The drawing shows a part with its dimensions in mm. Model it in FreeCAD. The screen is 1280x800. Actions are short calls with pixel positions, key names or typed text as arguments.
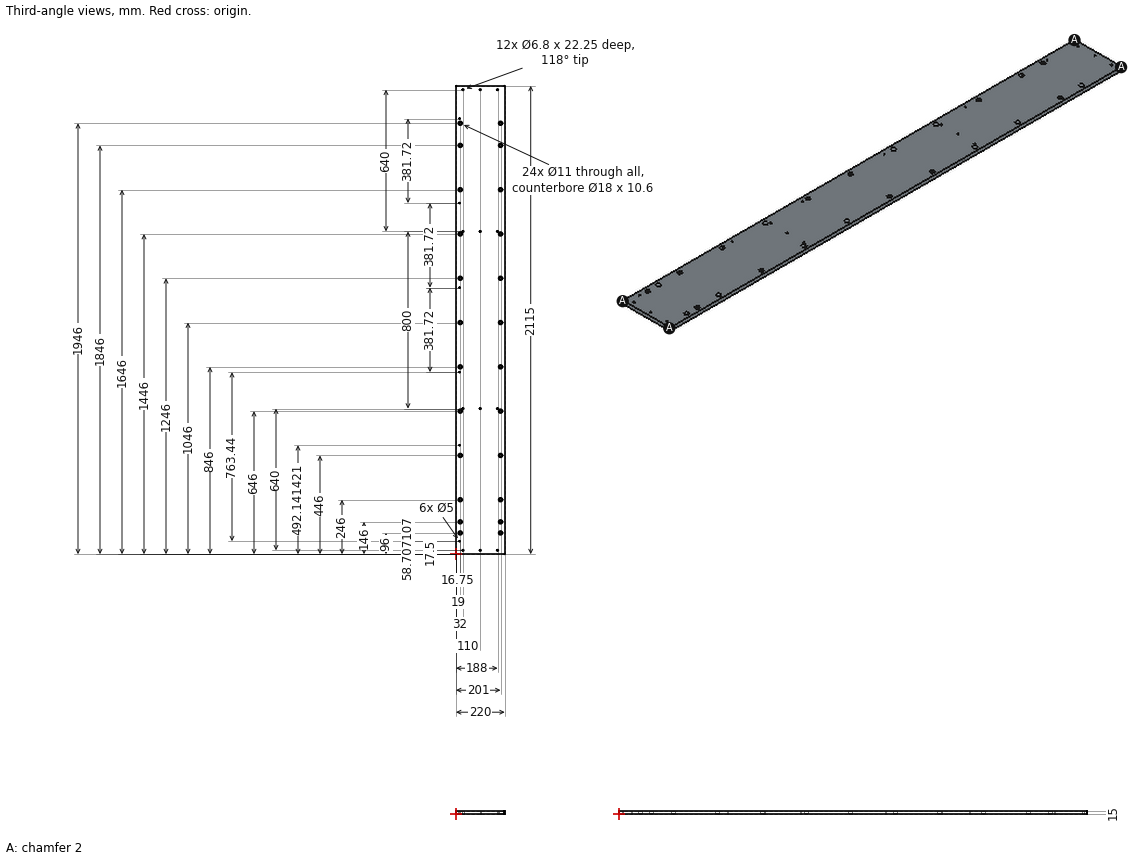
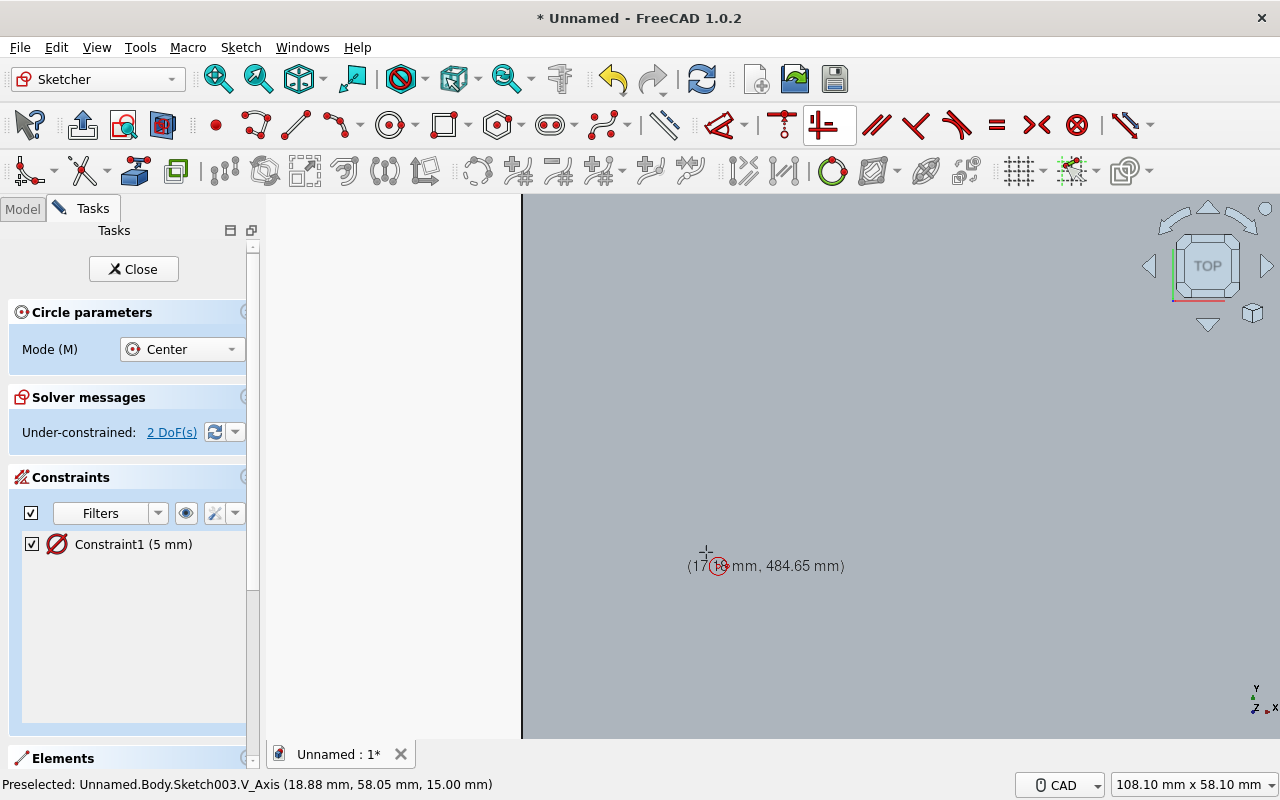
scroll(704, 466, down, 15)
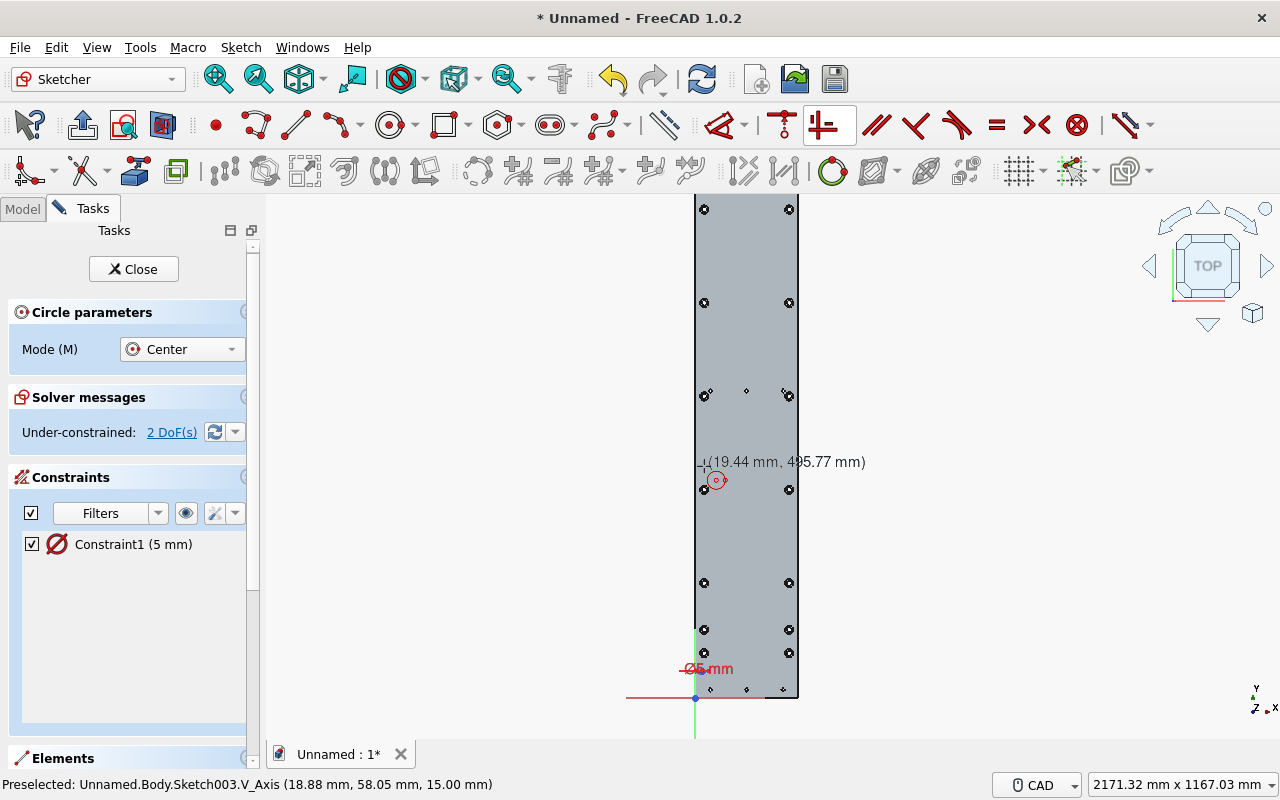
scroll(707, 599, down, 5)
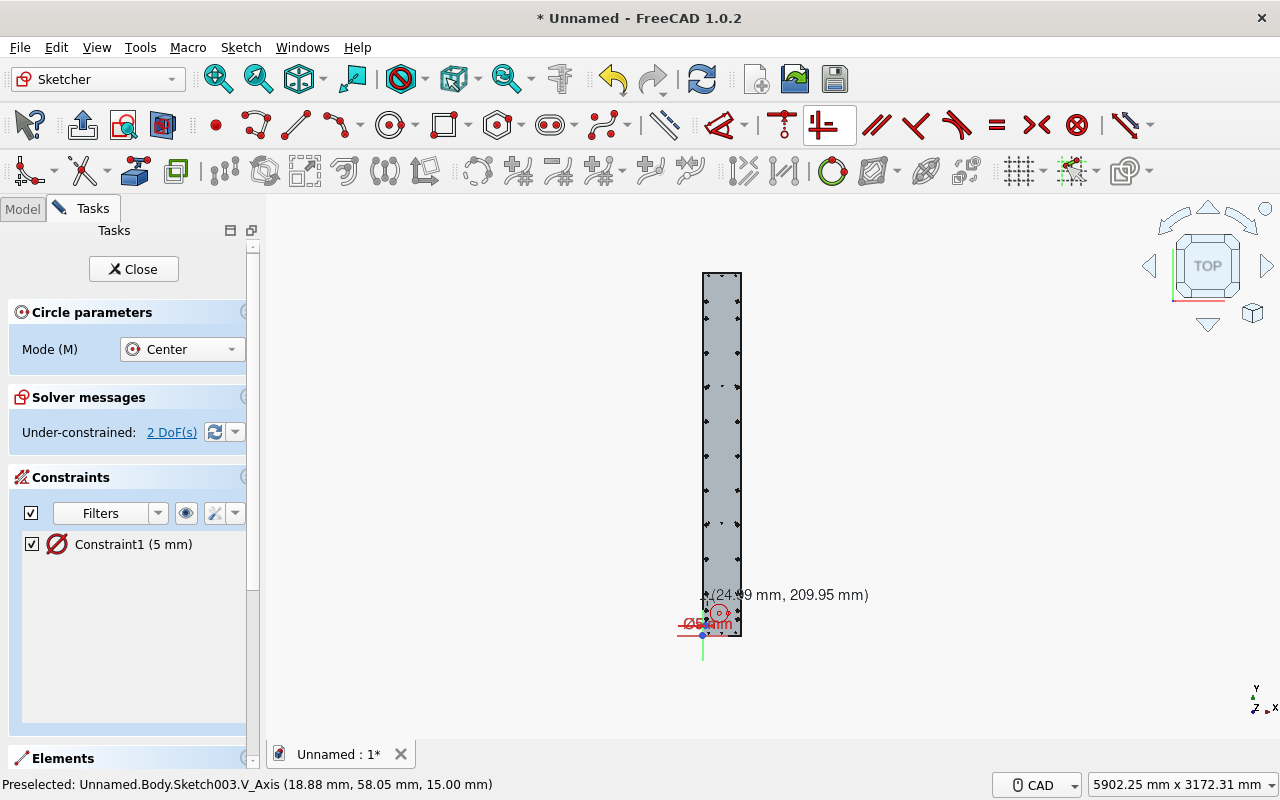
scroll(706, 551, up, 9)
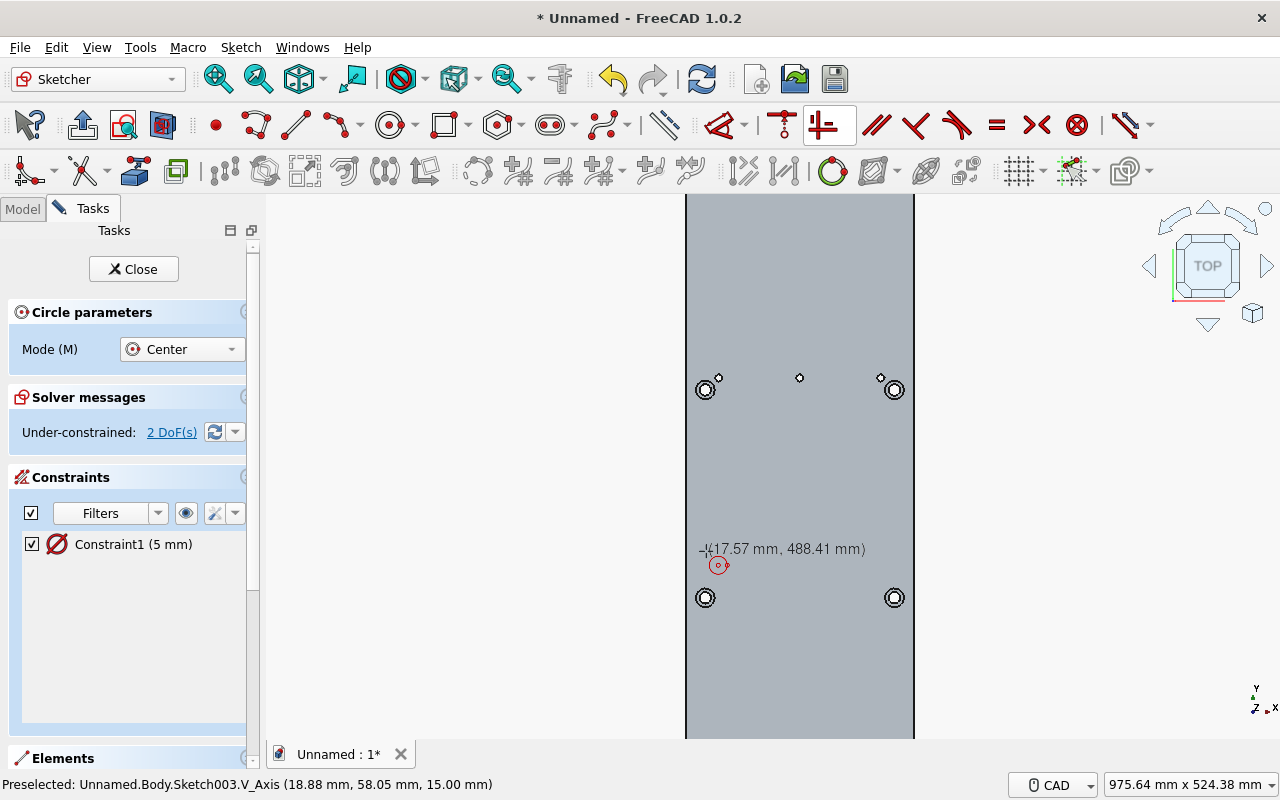
click(703, 550)
move(705, 548)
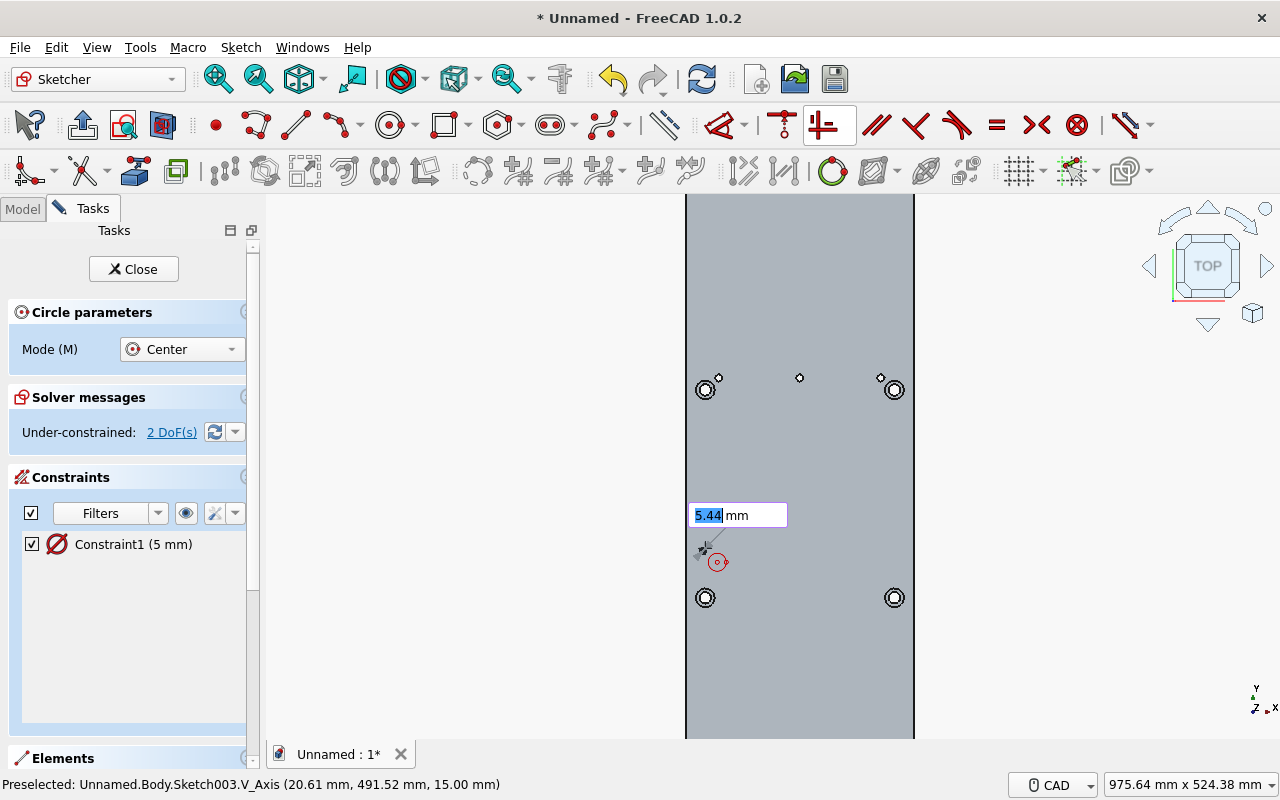
text(5)
key(Return)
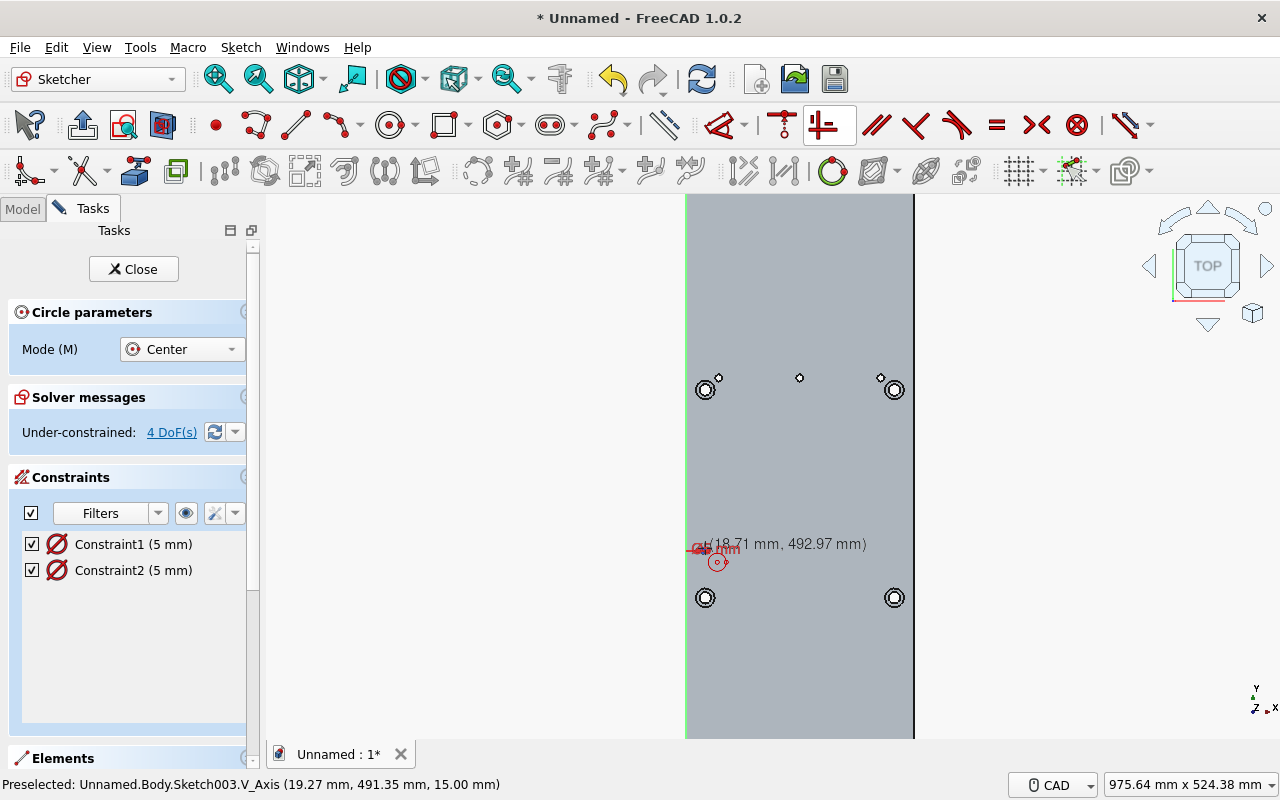
scroll(706, 551, down, 9)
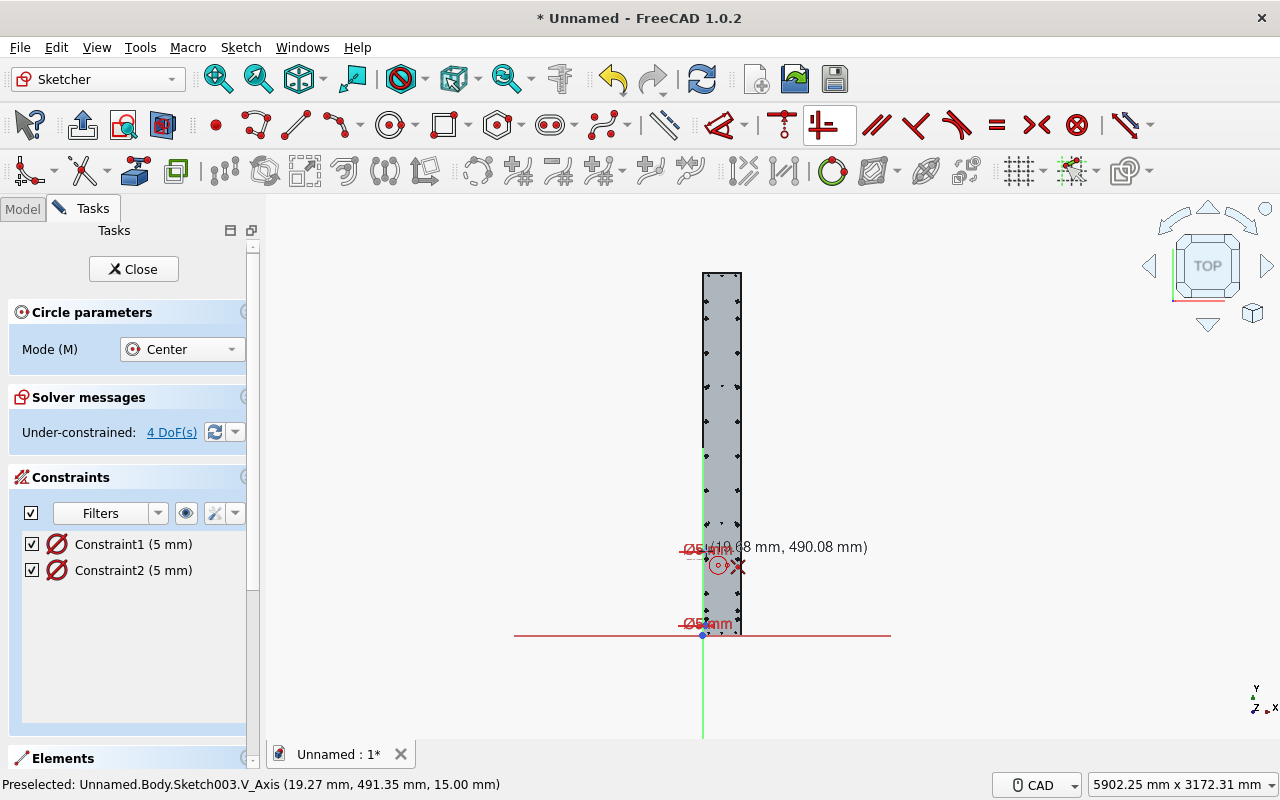
scroll(706, 495, up, 20)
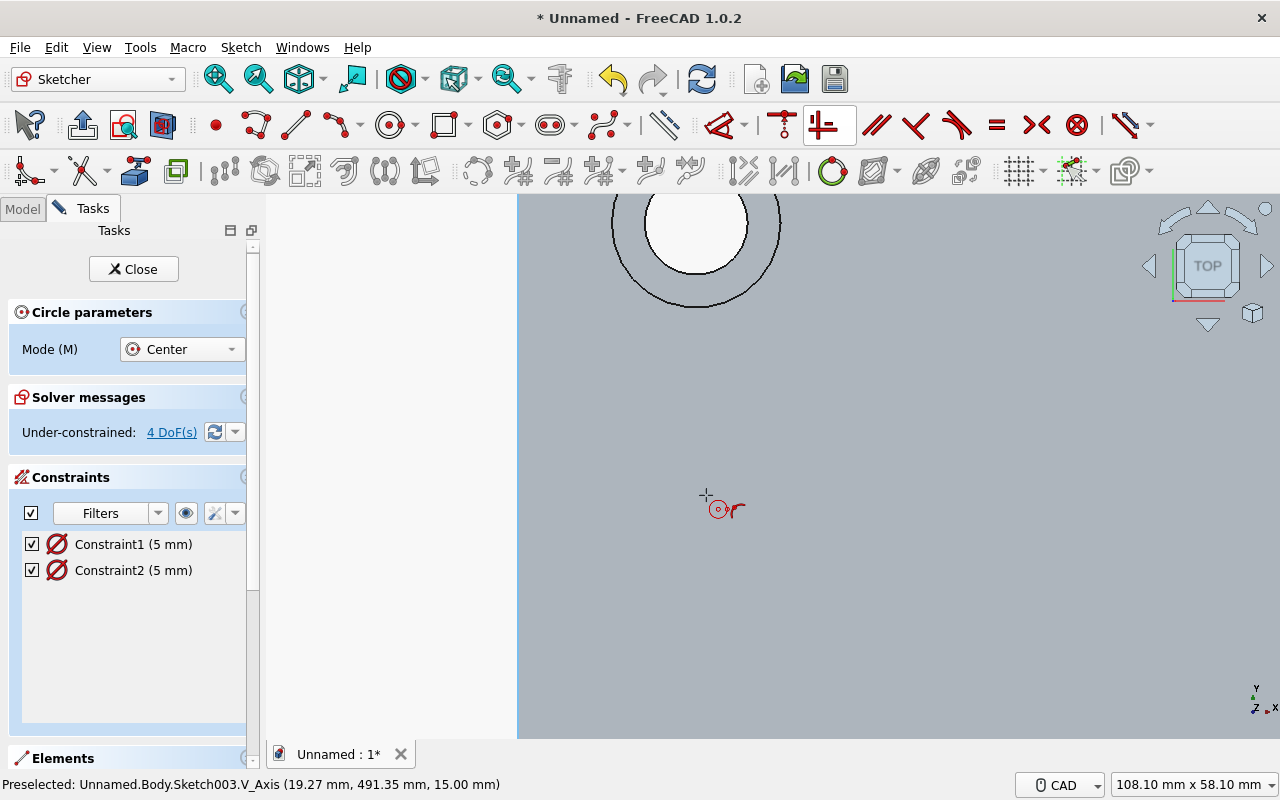
scroll(704, 466, down, 15)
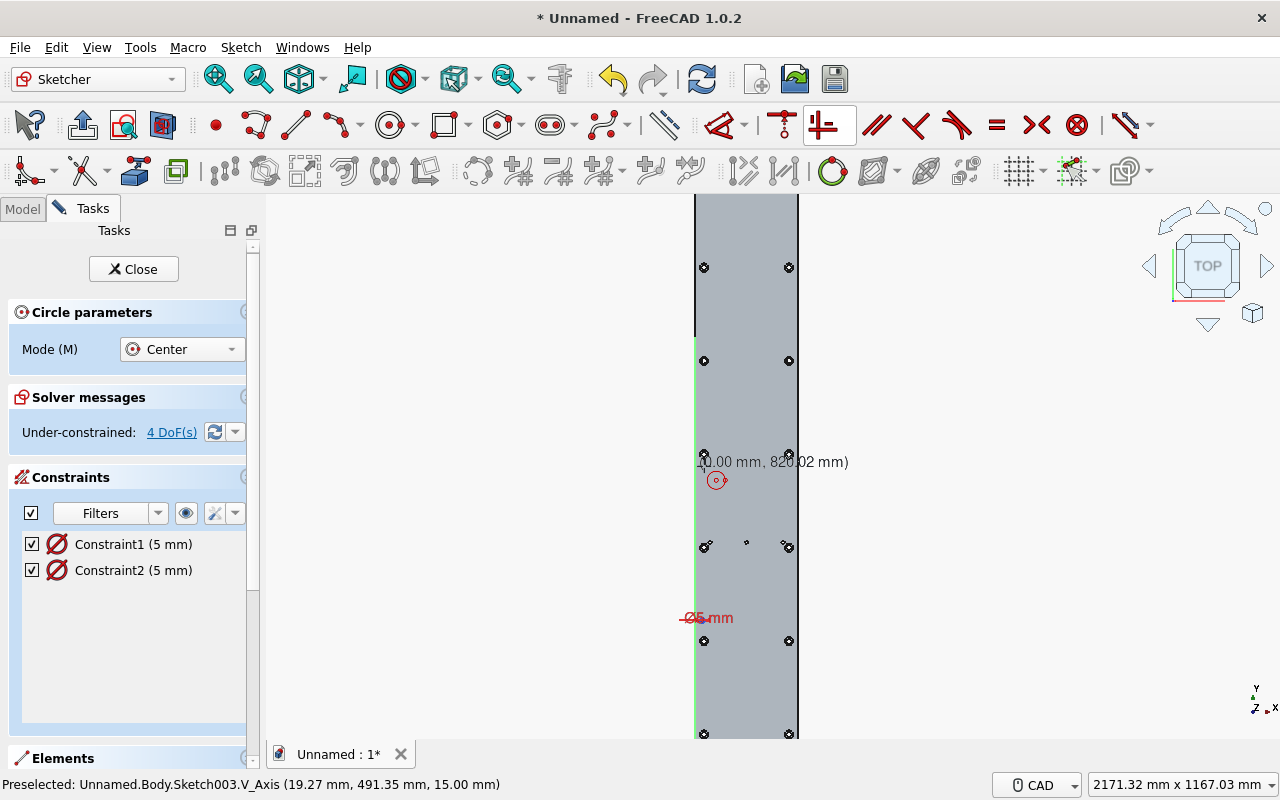
scroll(707, 511, down, 5)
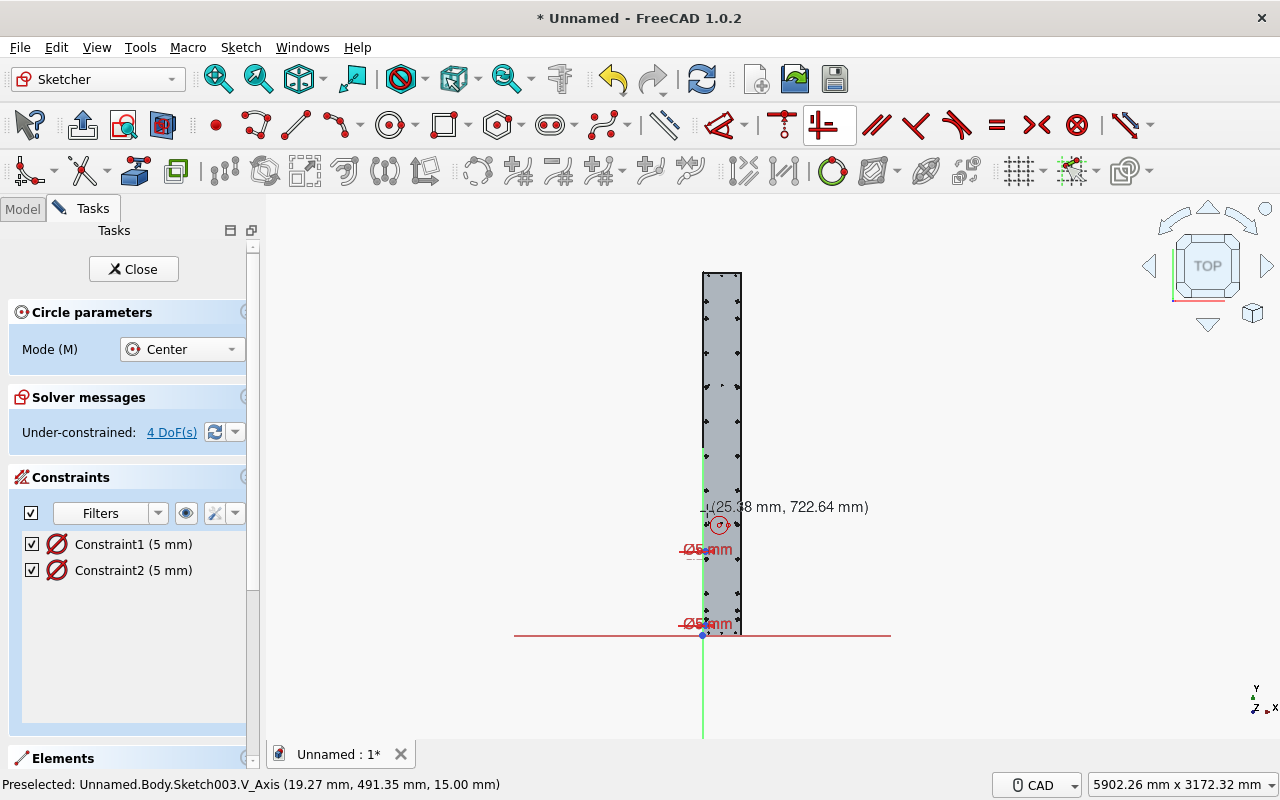
scroll(706, 495, up, 9)